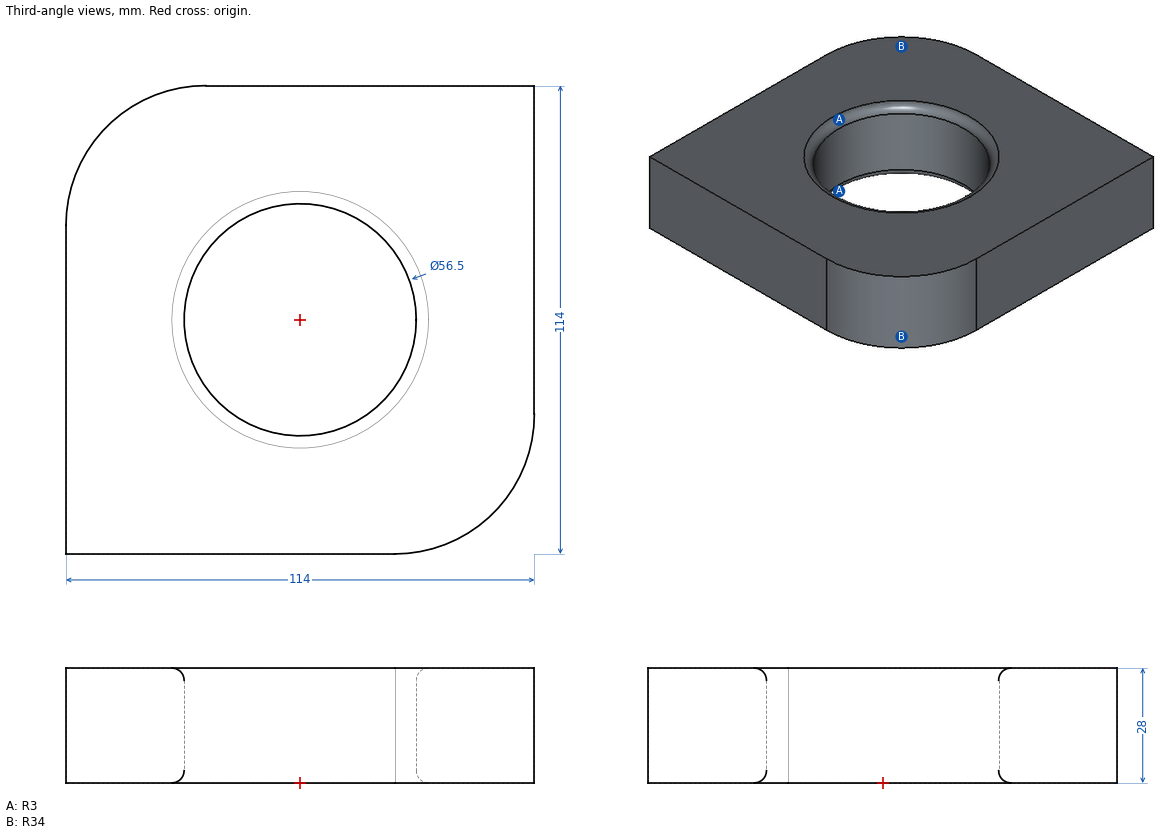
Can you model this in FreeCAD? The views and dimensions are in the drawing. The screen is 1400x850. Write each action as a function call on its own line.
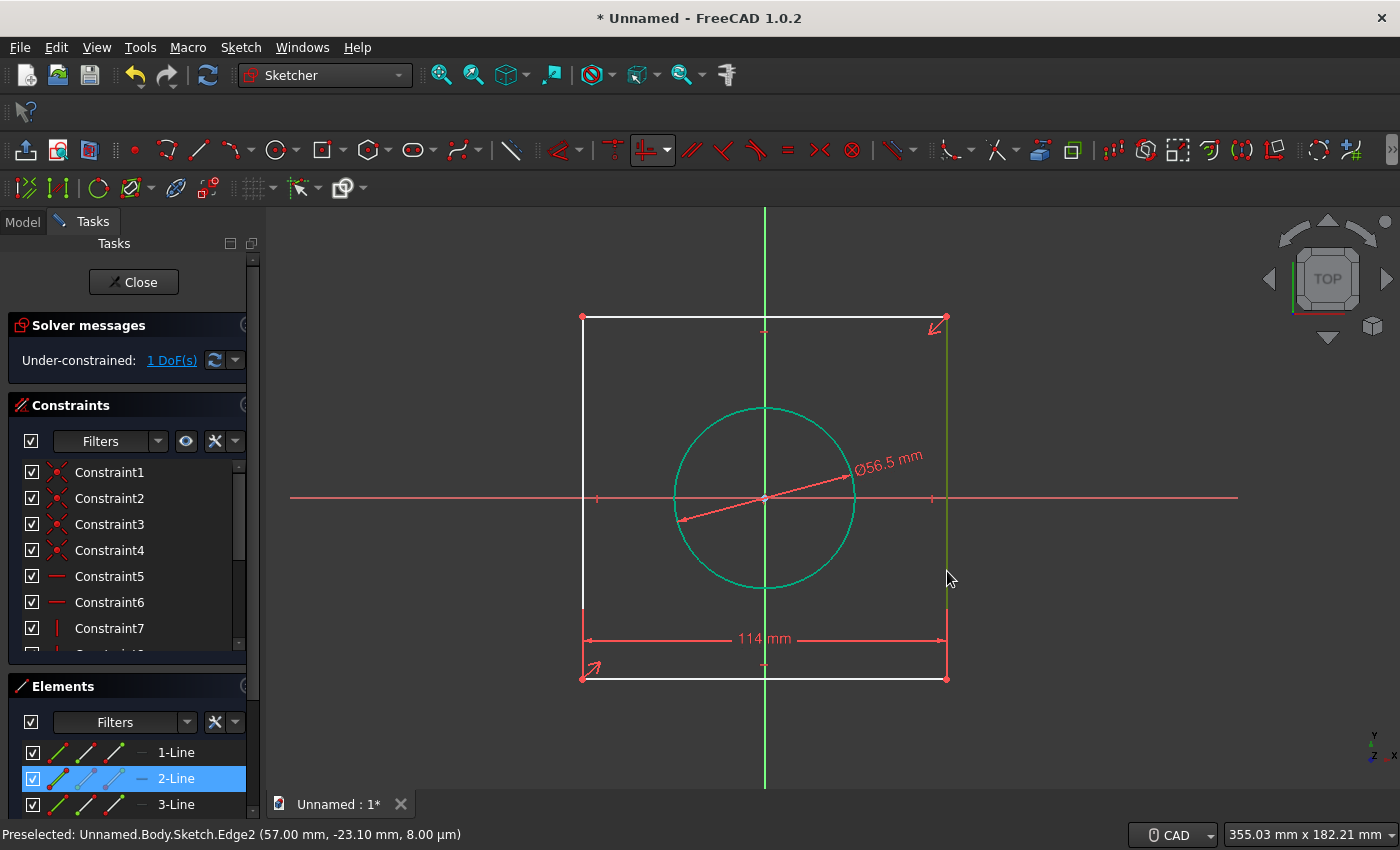
click(582, 150)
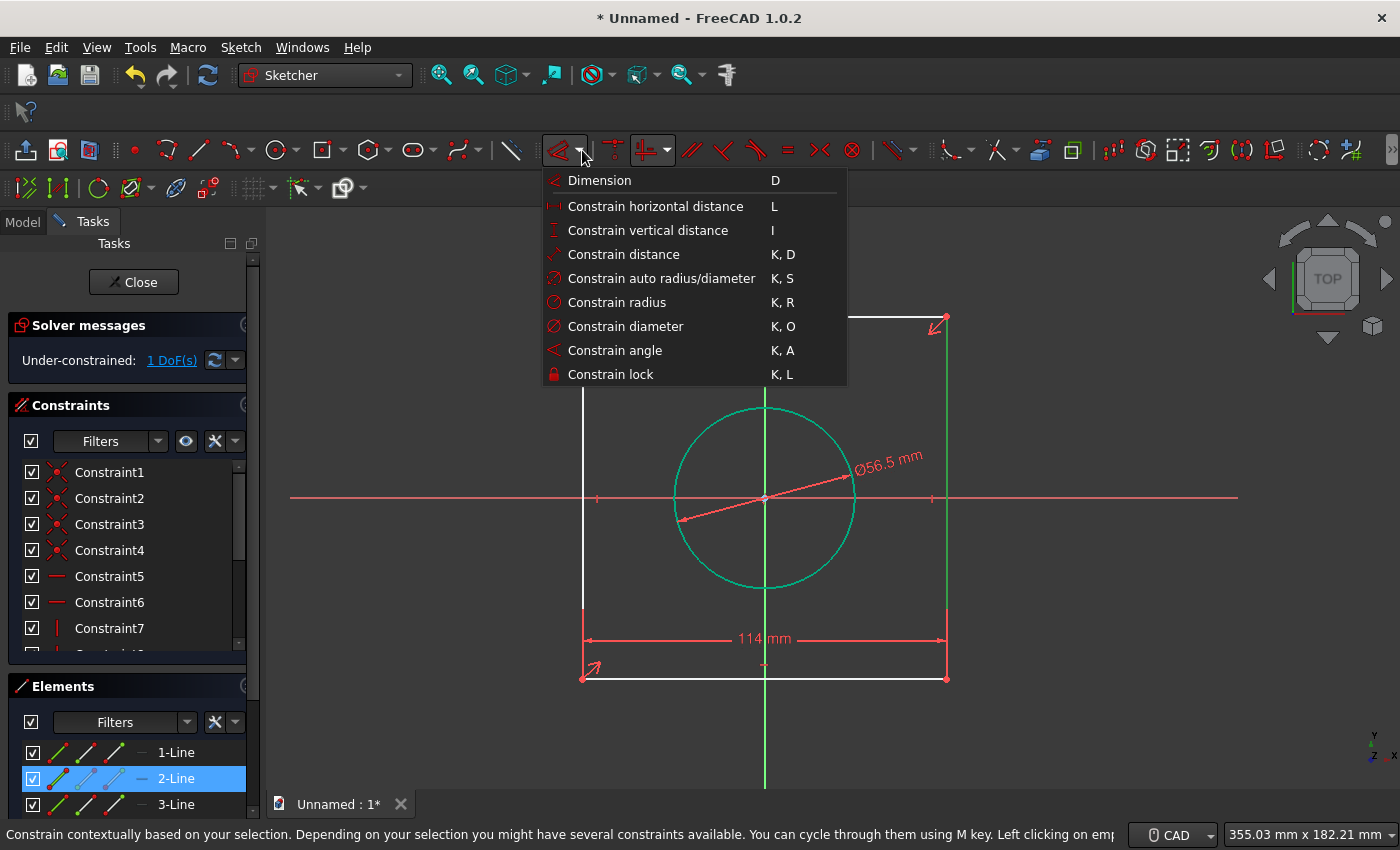
click(695, 230)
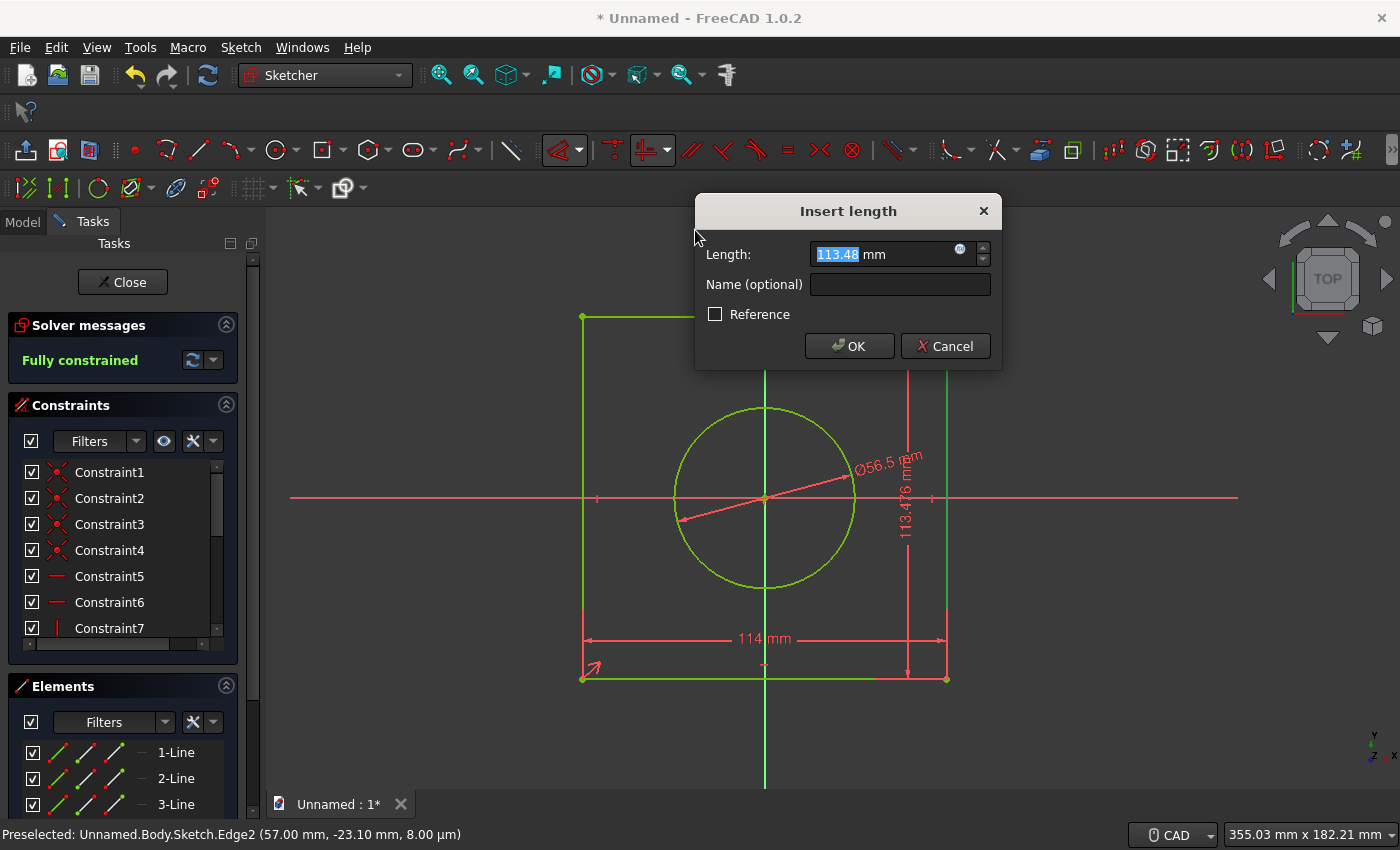
text(114)
key(Return)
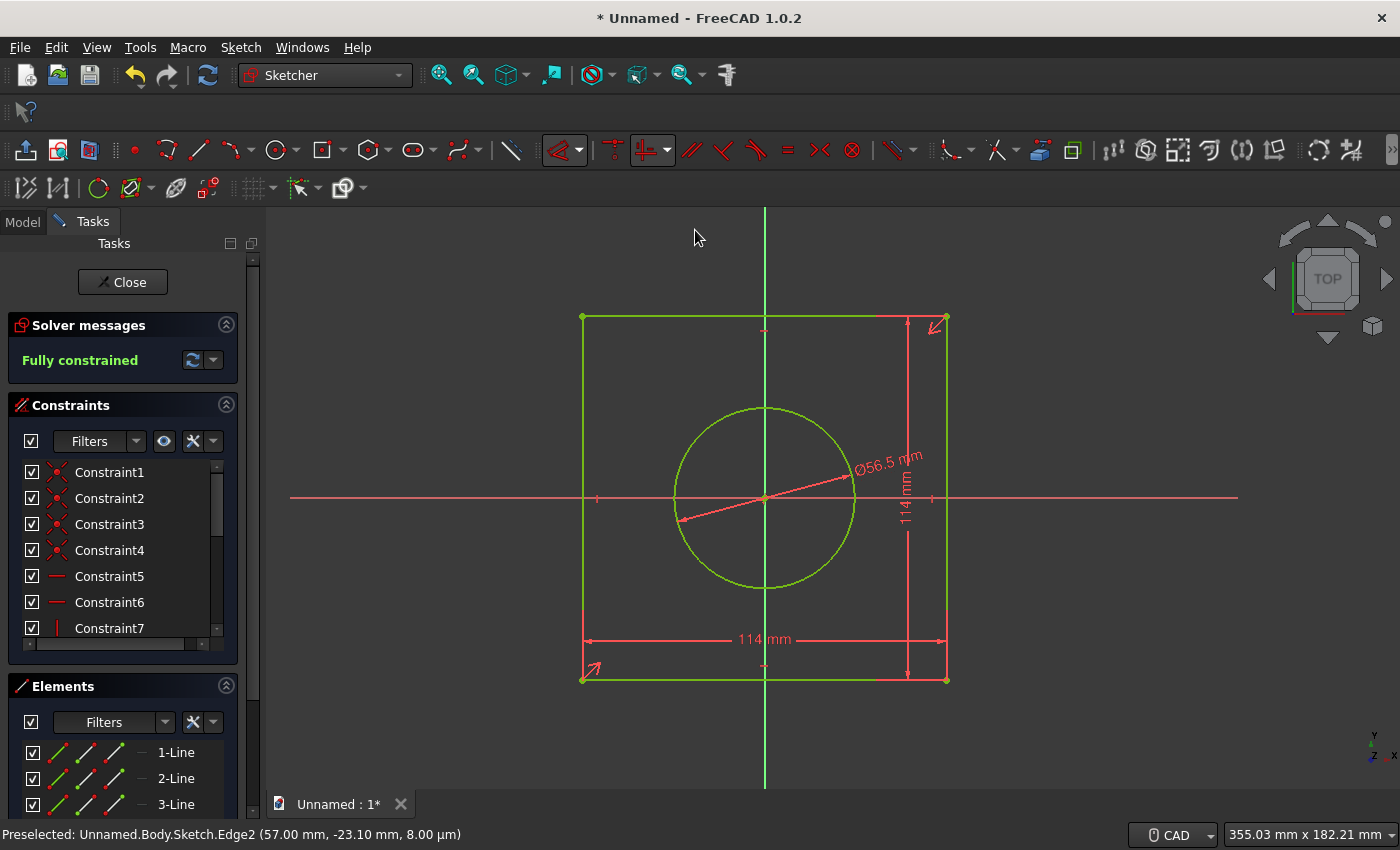
click(123, 282)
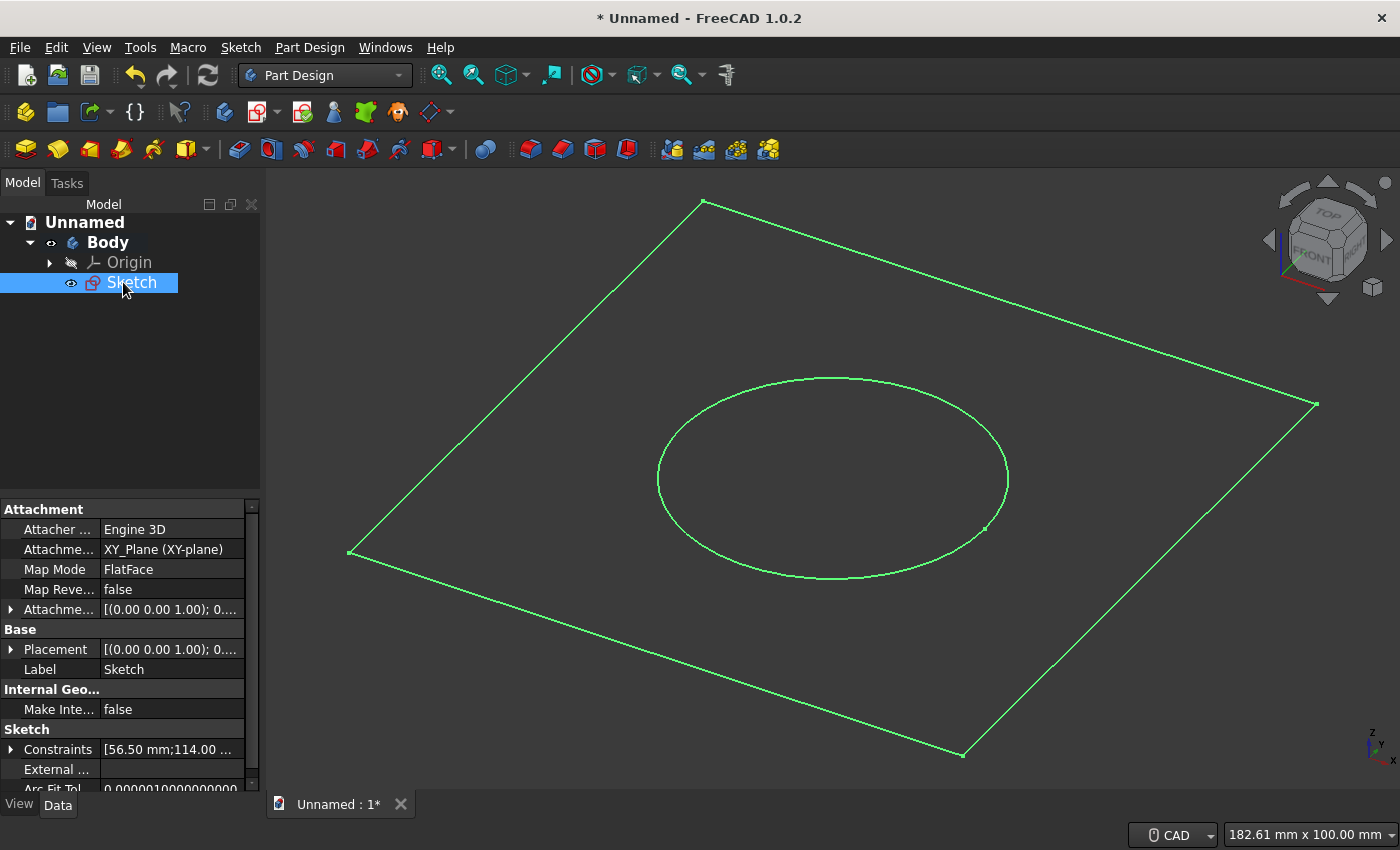
click(26, 150)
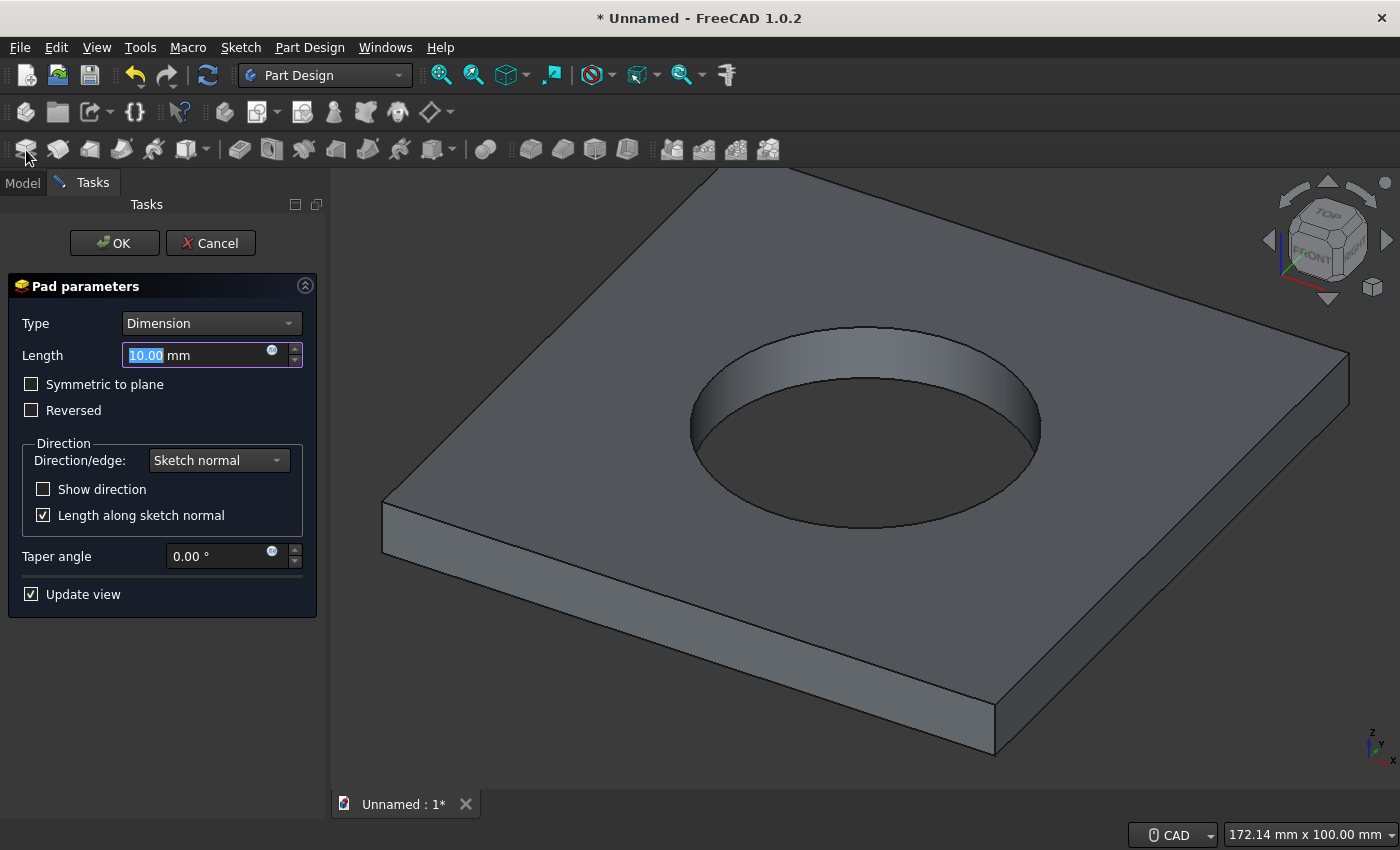
text(28)
key(Tab)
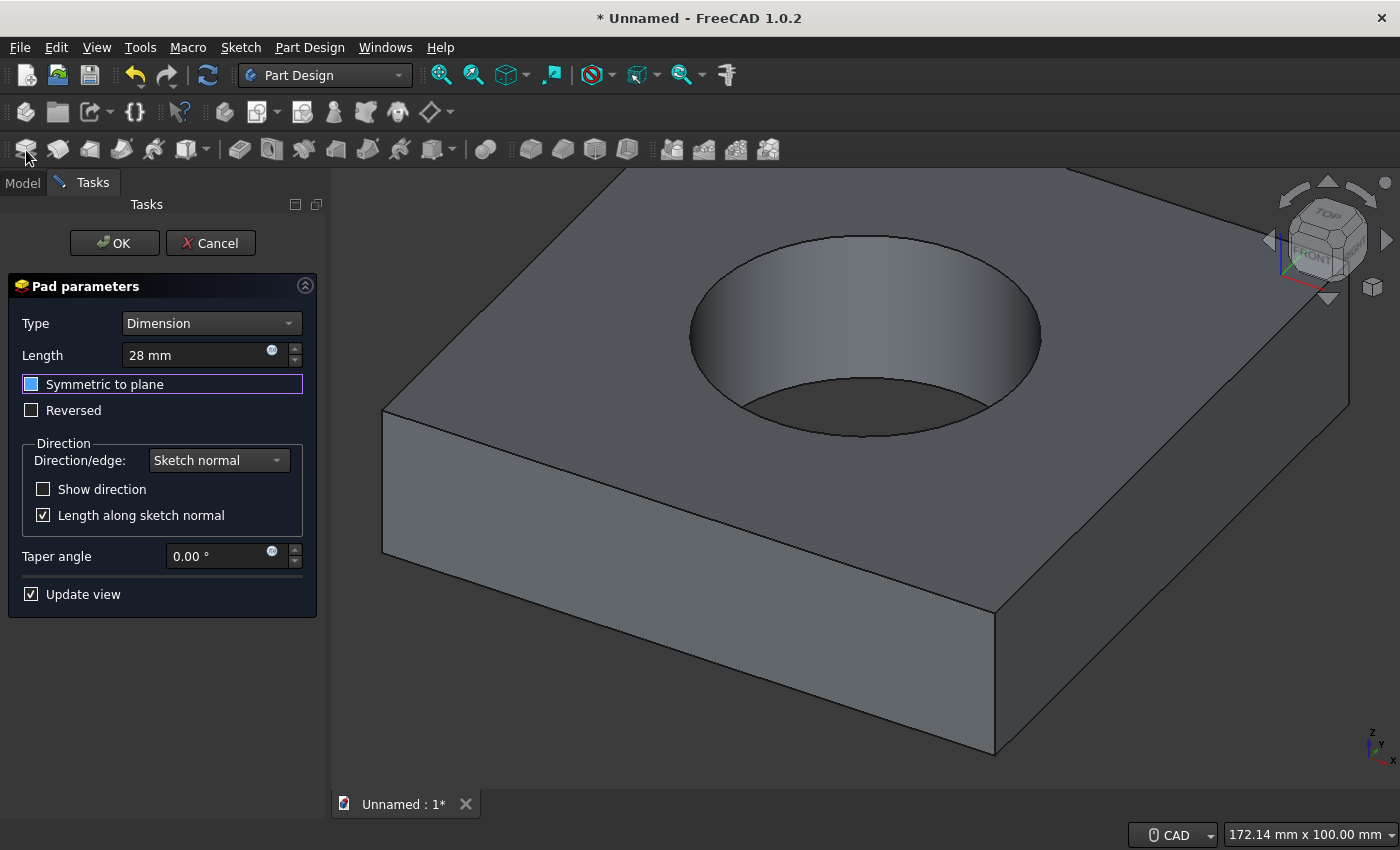
click(115, 243)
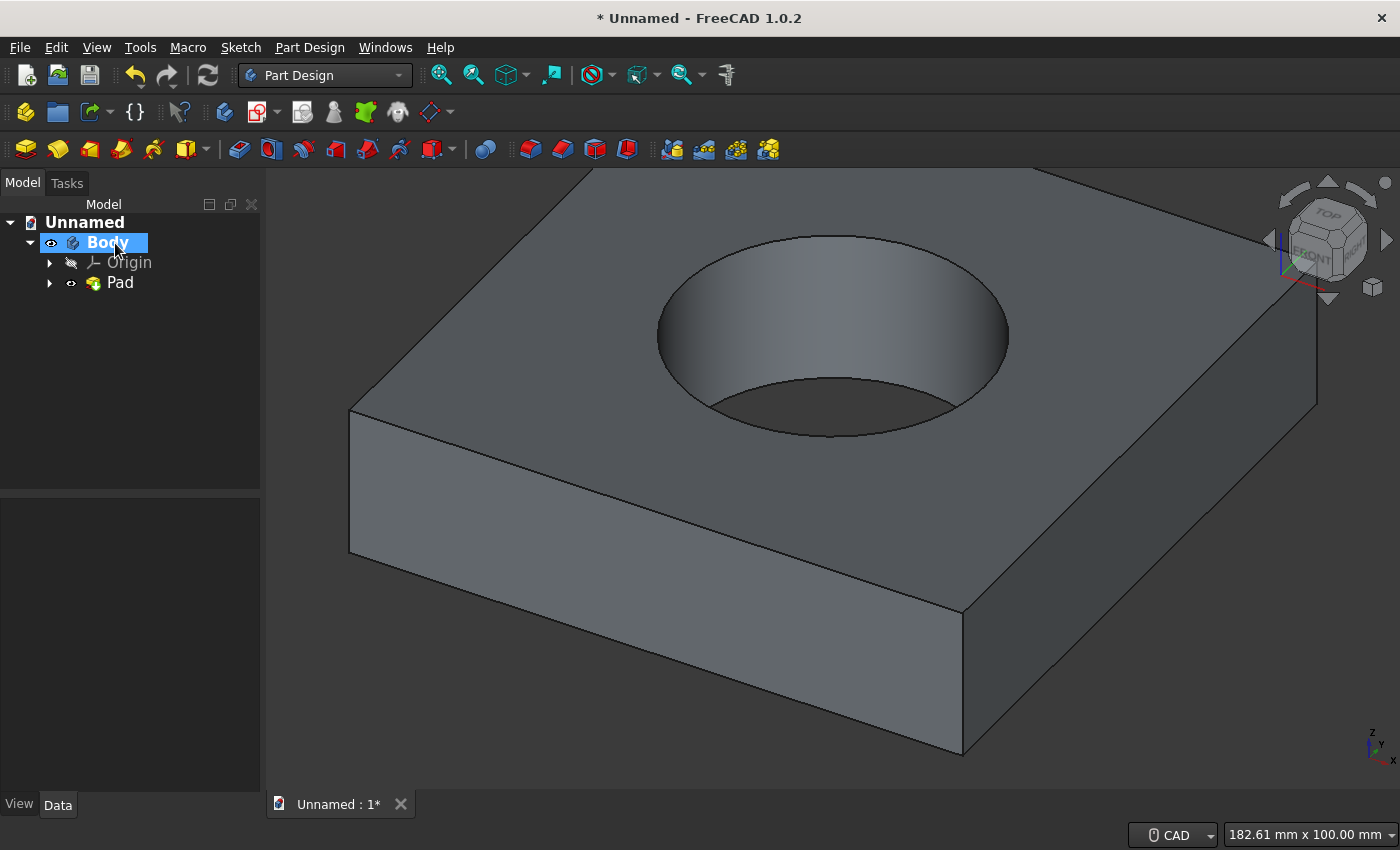
key(v)
key(f)